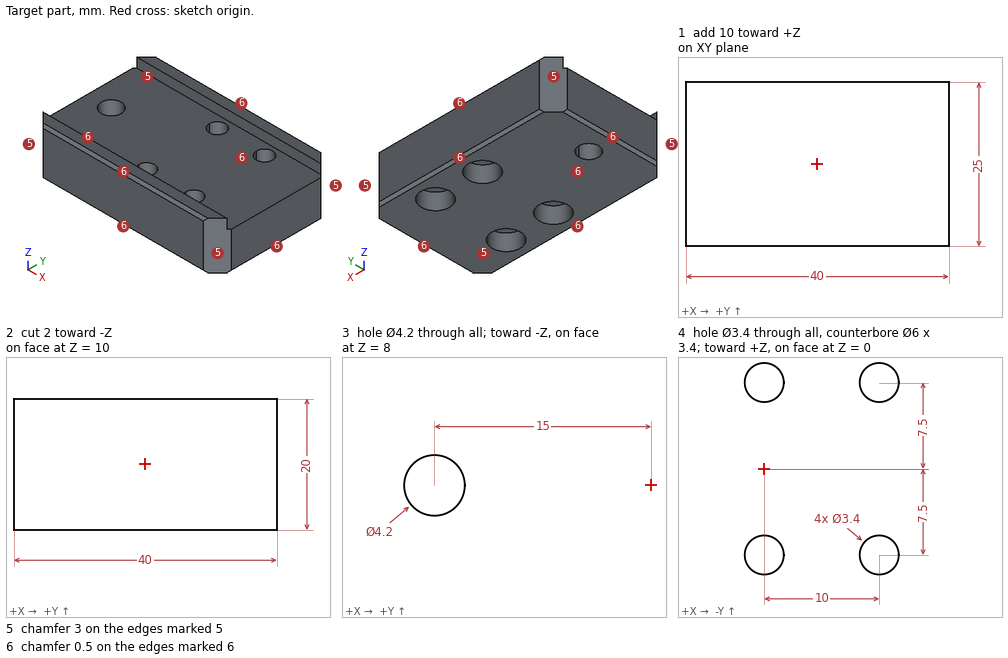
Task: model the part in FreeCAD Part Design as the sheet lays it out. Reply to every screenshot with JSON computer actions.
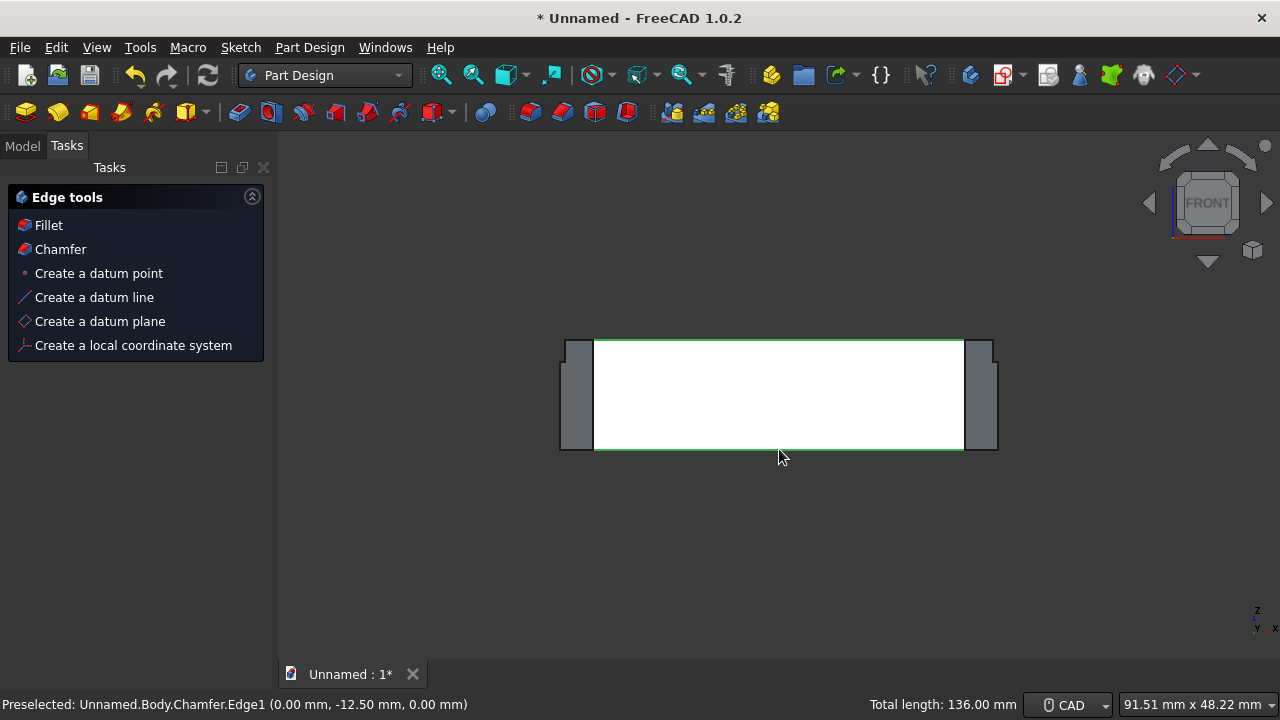
{"action": "key", "text": "3"}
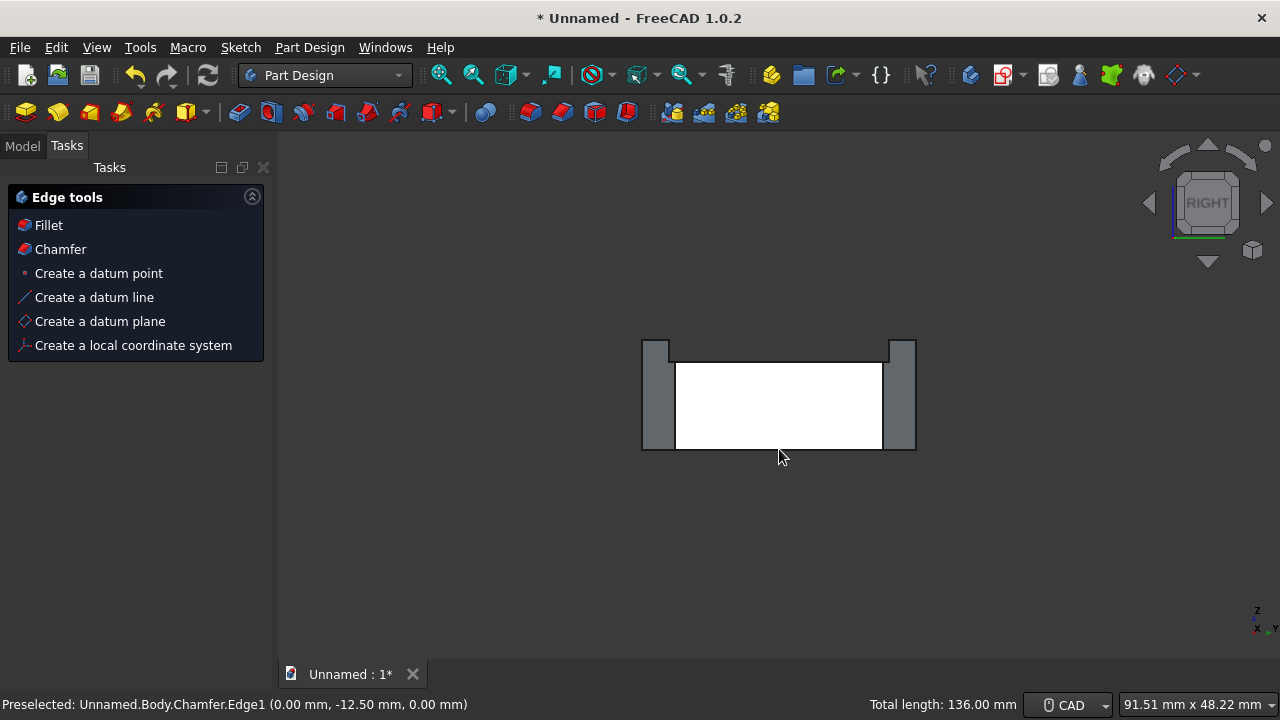
{"action": "left_click", "coordinate": [442, 76]}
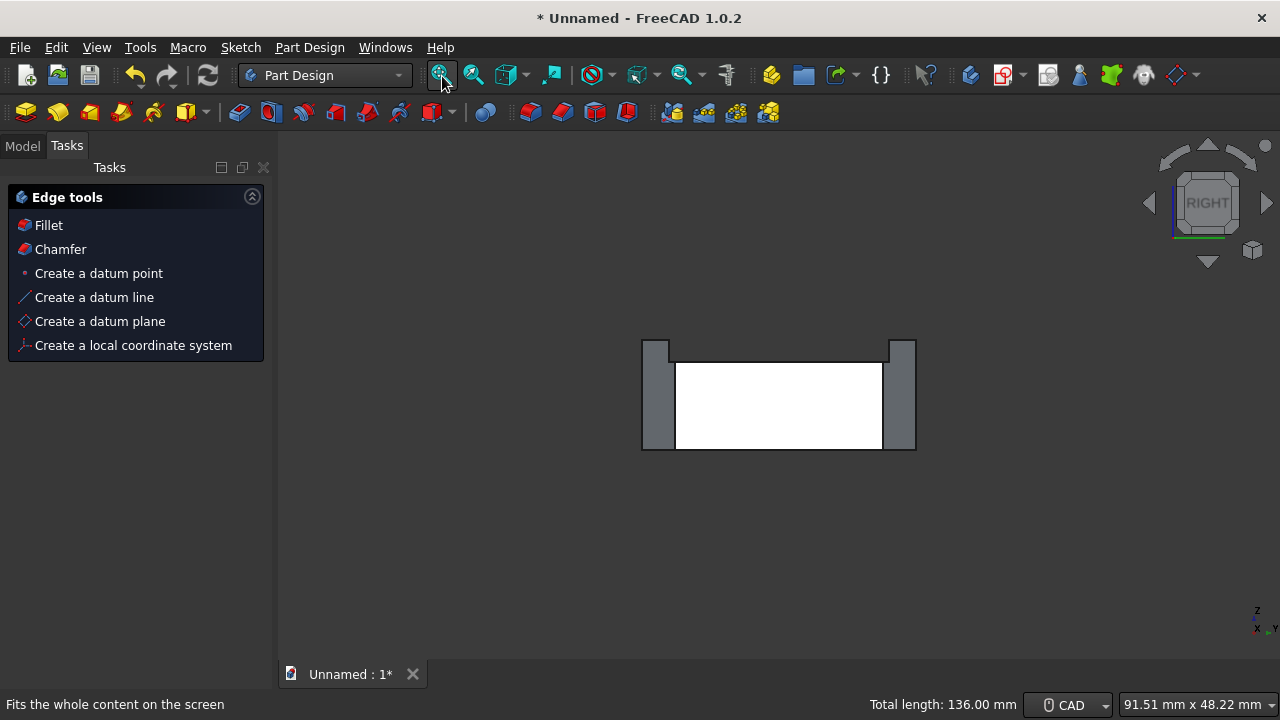
{"action": "left_click", "coordinate": [779, 449], "text": "ctrl"}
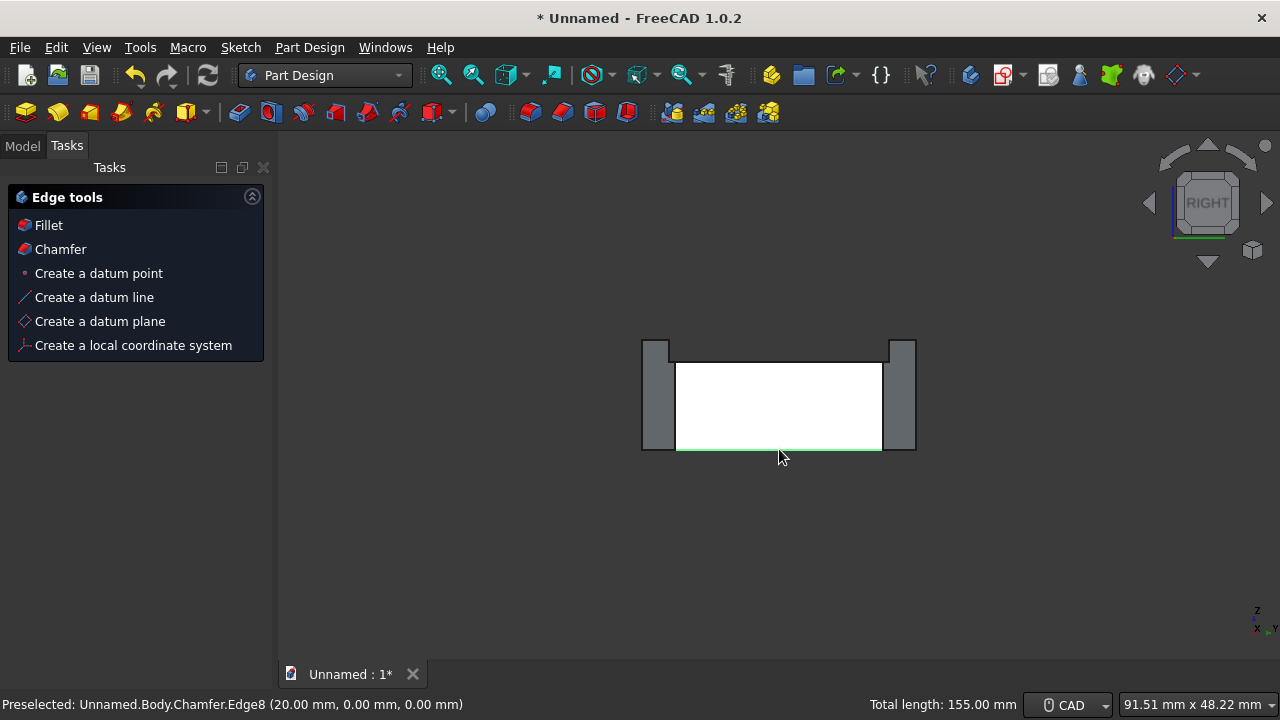
{"action": "key", "text": "5"}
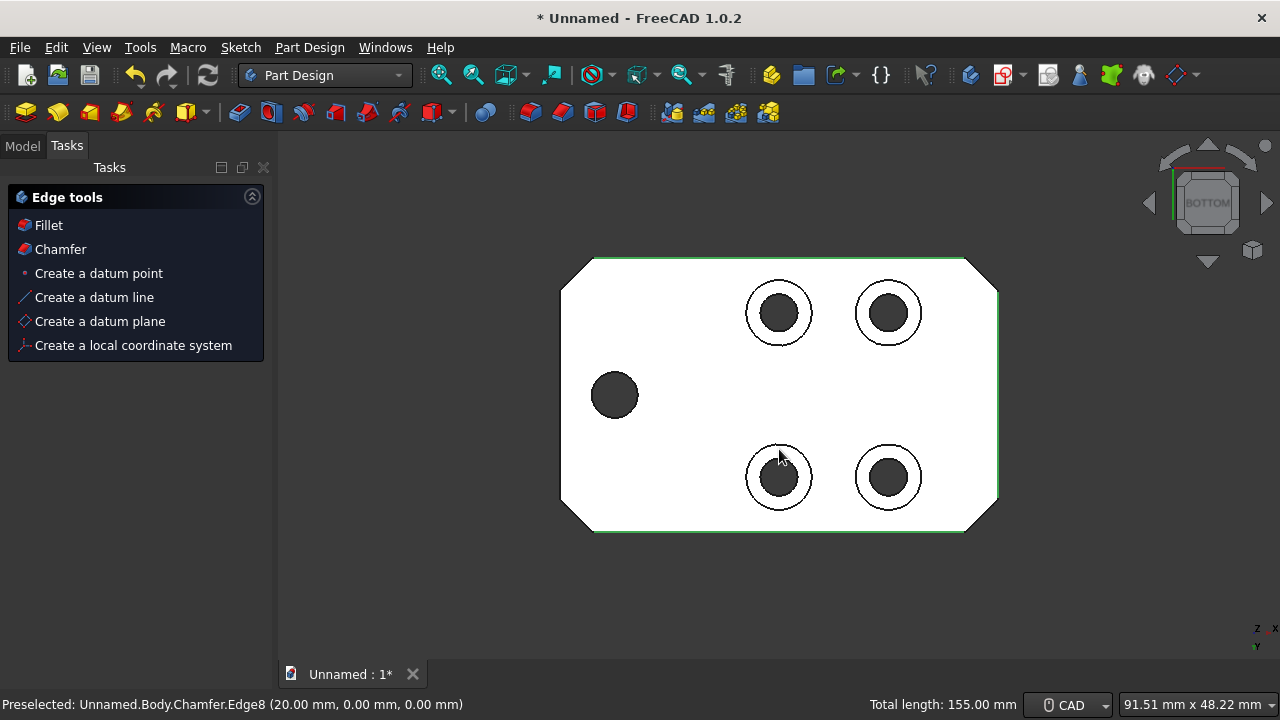
{"action": "left_click", "coordinate": [560, 394], "text": "ctrl"}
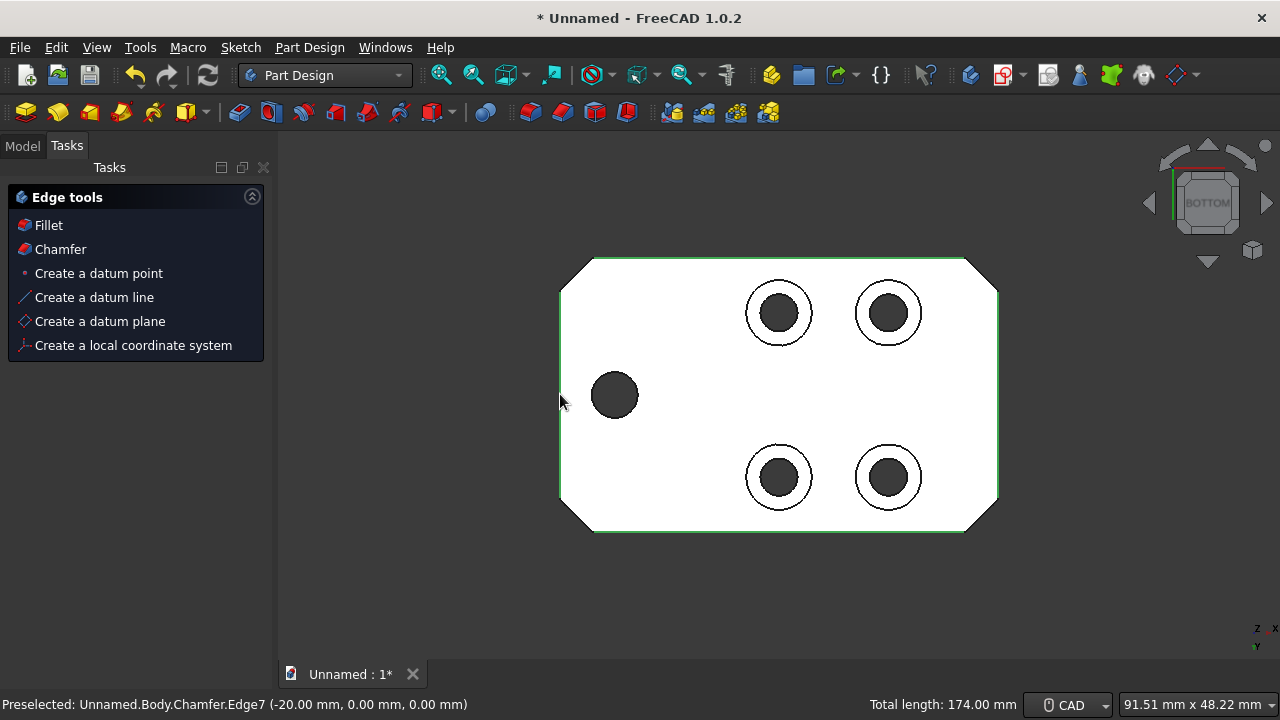
{"action": "left_click", "coordinate": [564, 112]}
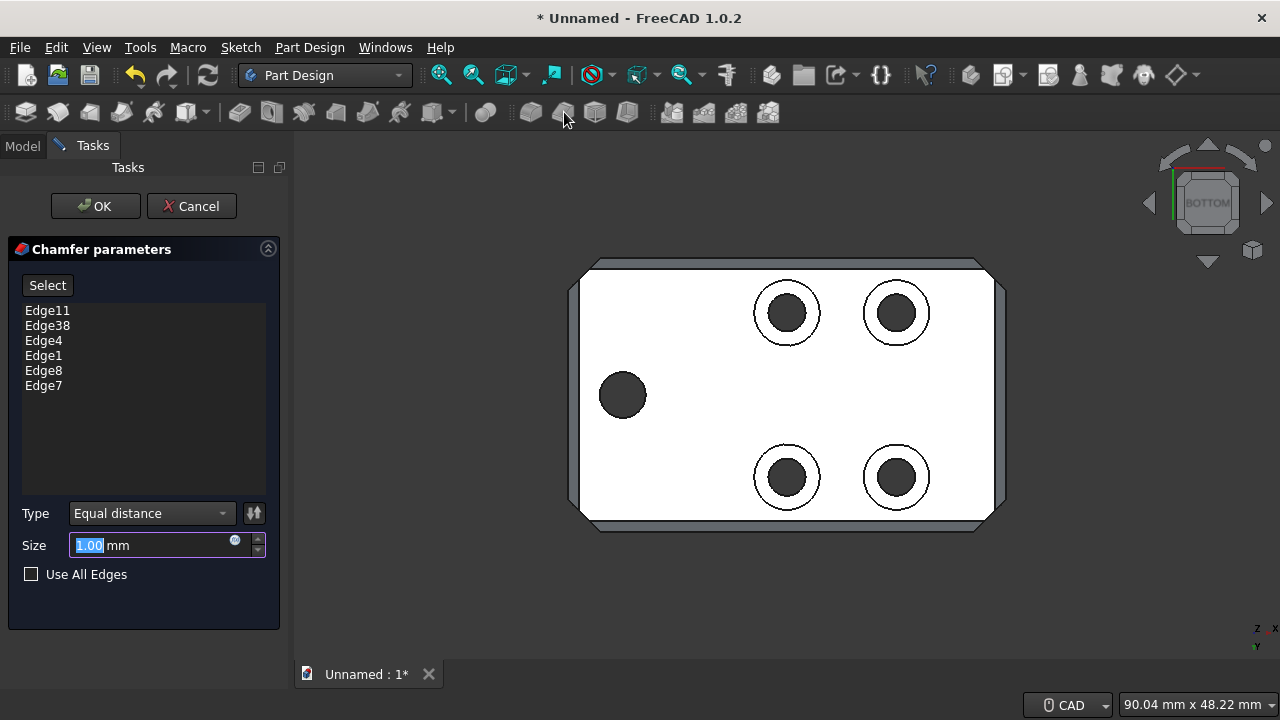
{"action": "type", "text": "0.5"}
{"action": "key", "text": "Tab"}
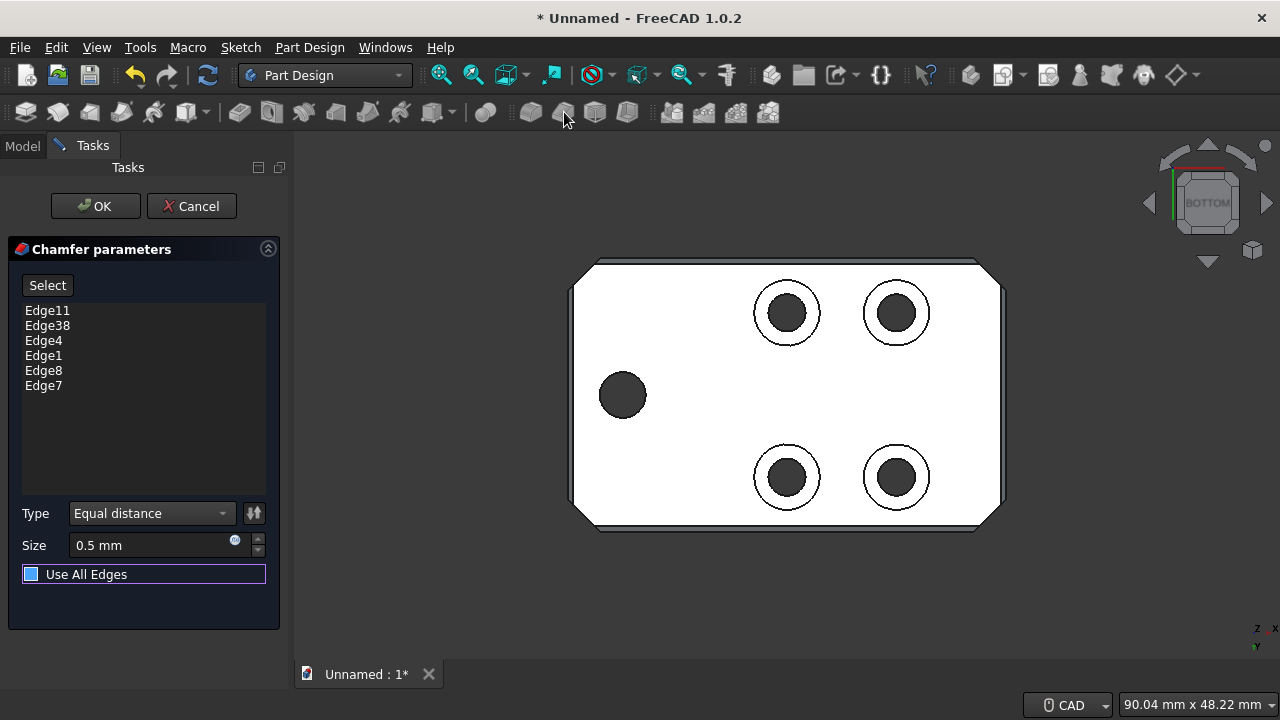
{"action": "left_click", "coordinate": [96, 206]}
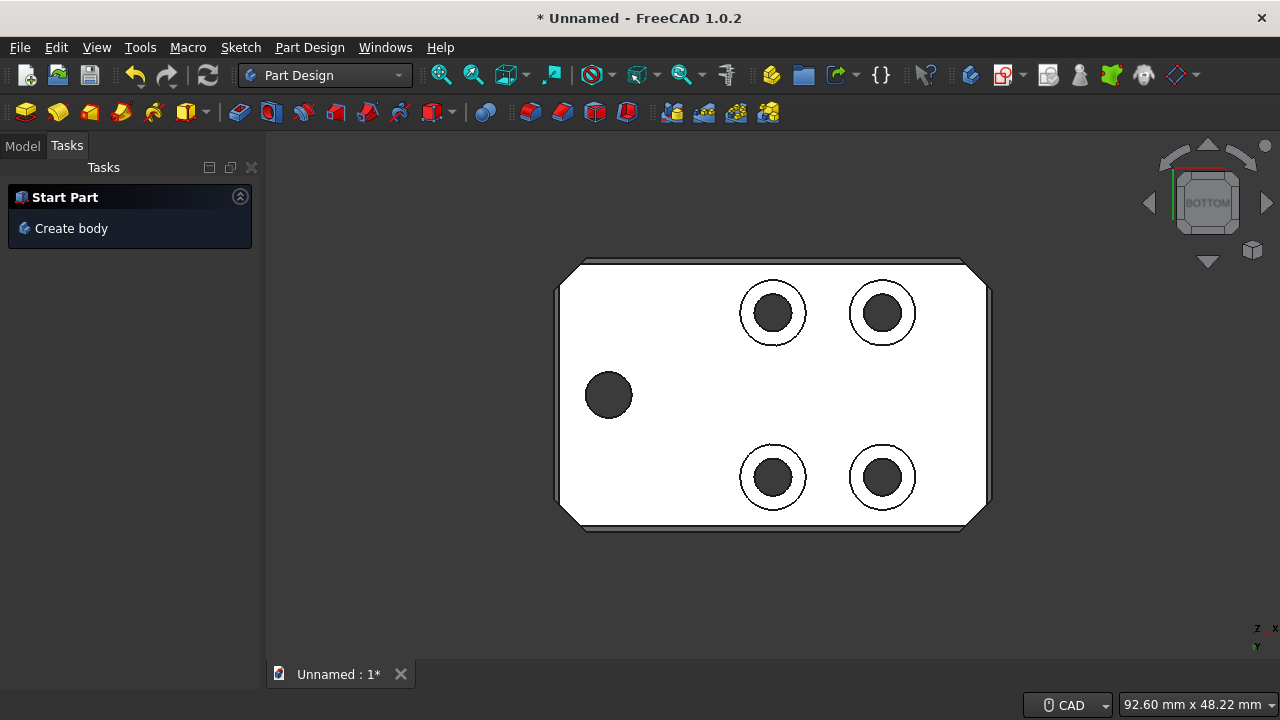
{"action": "key", "text": "0"}